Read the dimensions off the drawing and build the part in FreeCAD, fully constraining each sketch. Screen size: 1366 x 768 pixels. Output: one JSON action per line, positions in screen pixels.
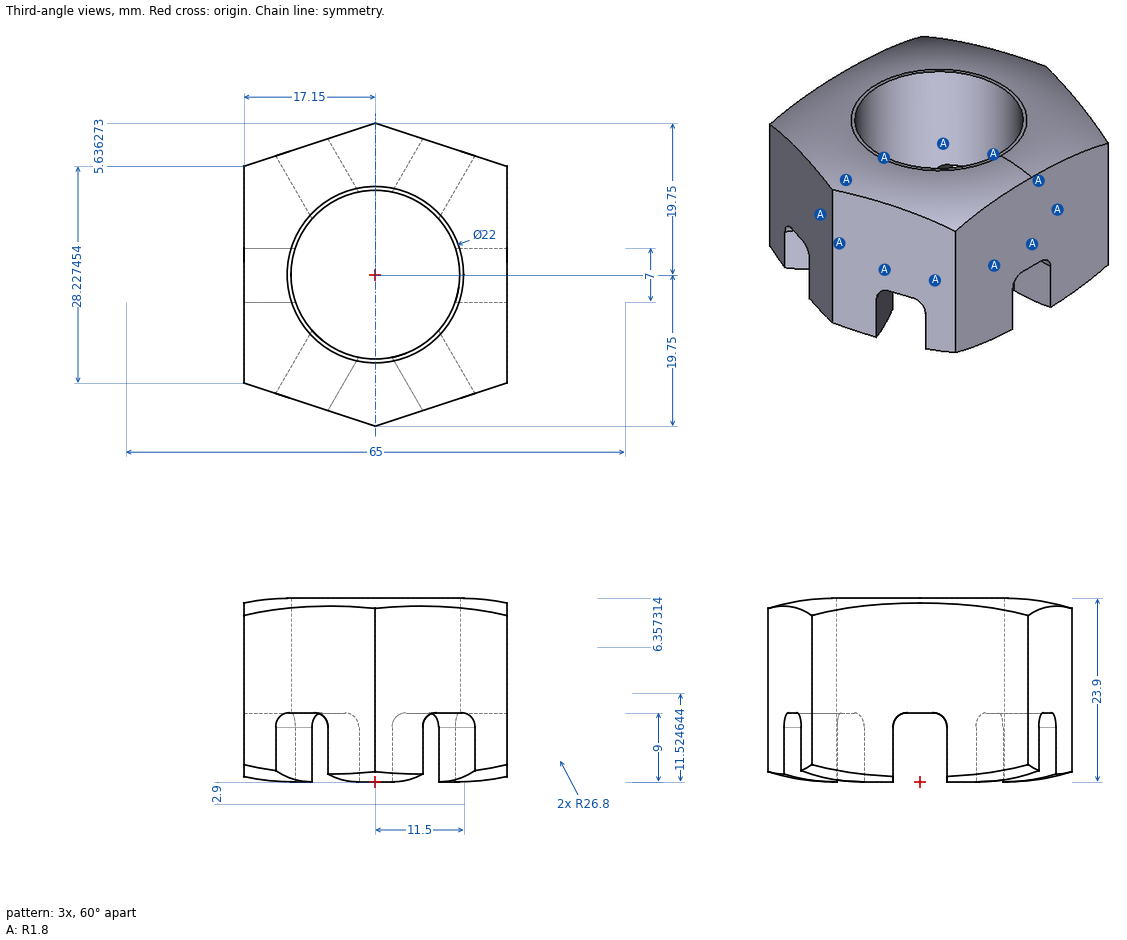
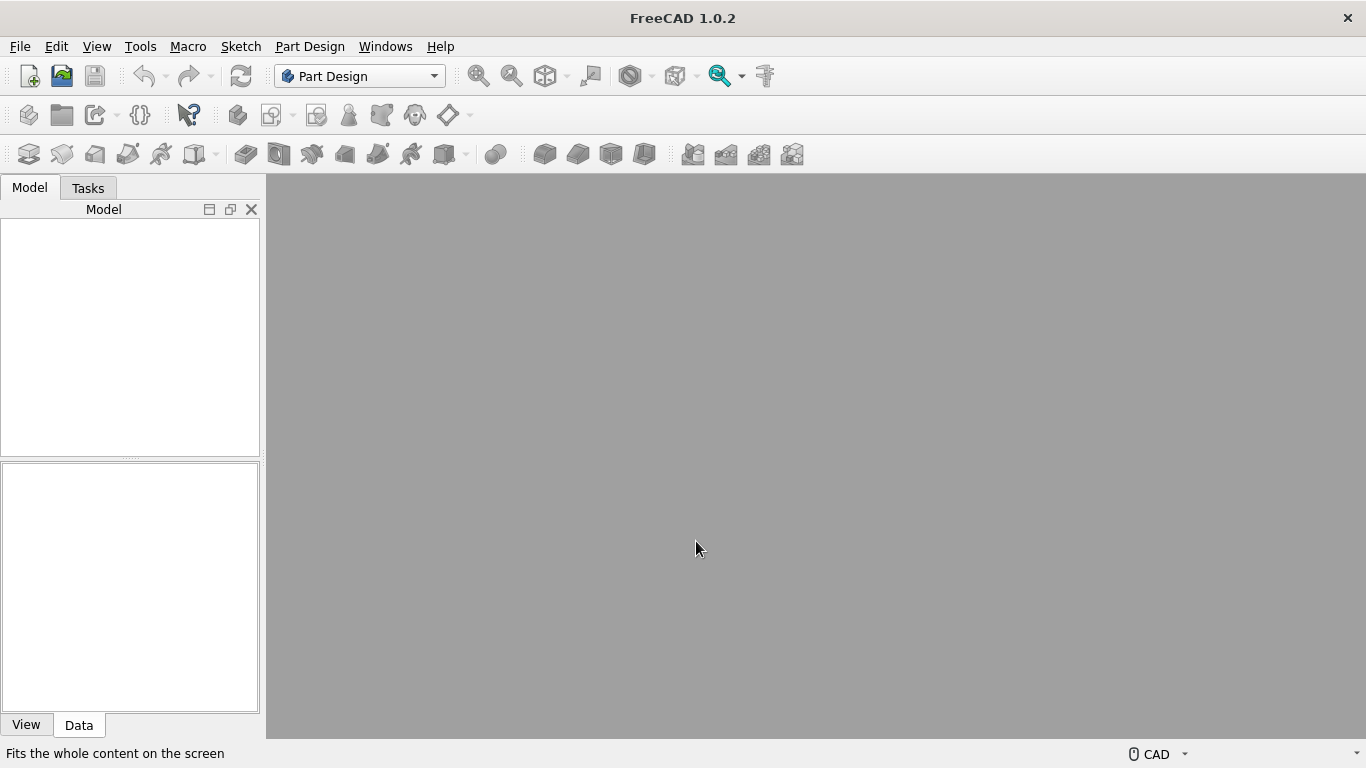
{"action": "left_click", "coordinate": [29, 76]}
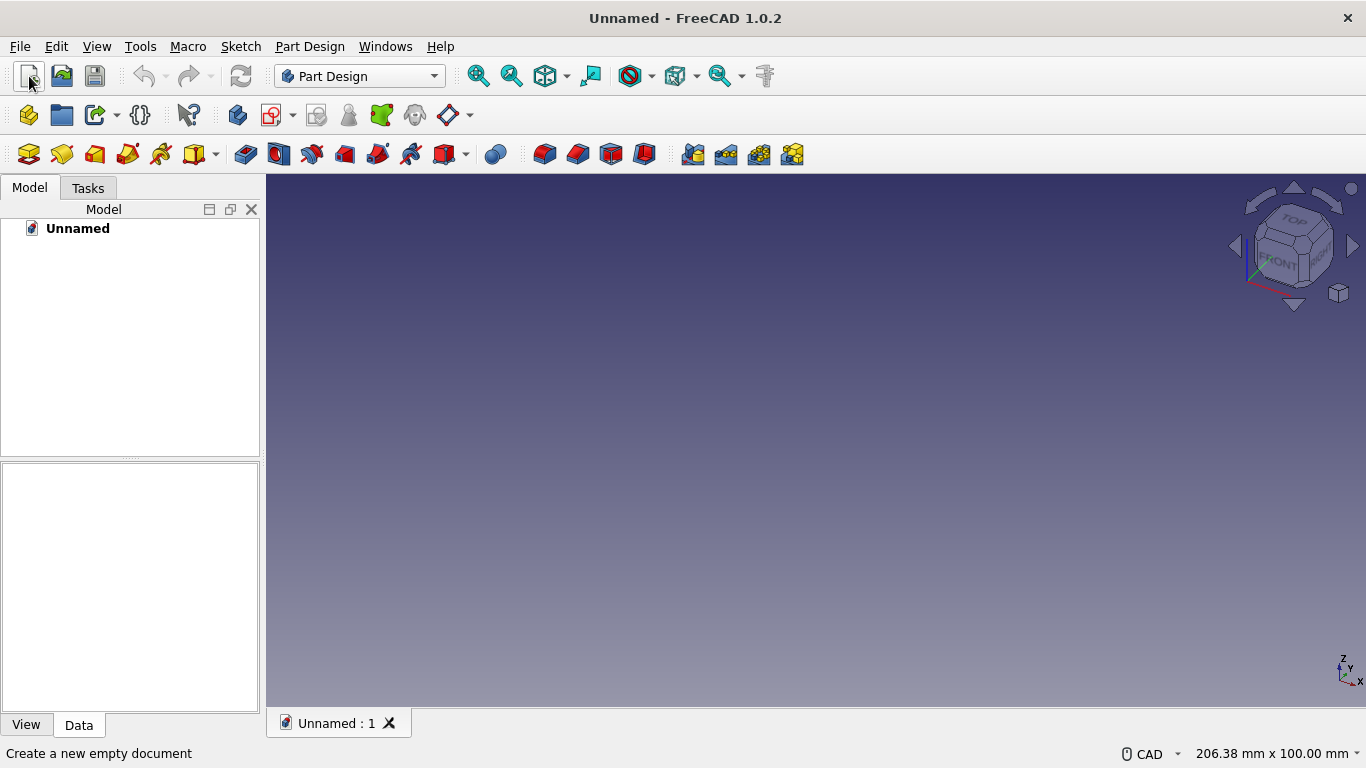
{"action": "left_click", "coordinate": [270, 116]}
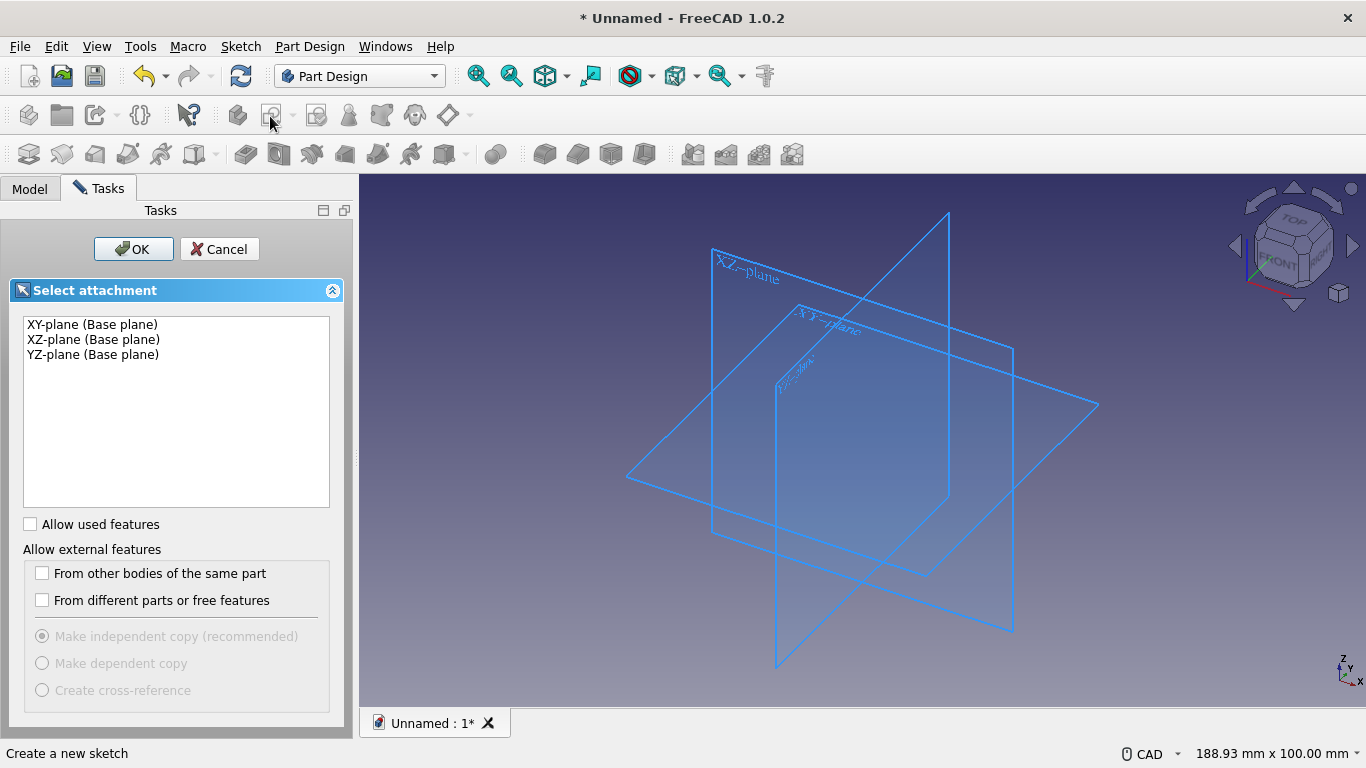
{"action": "left_click", "coordinate": [84, 324]}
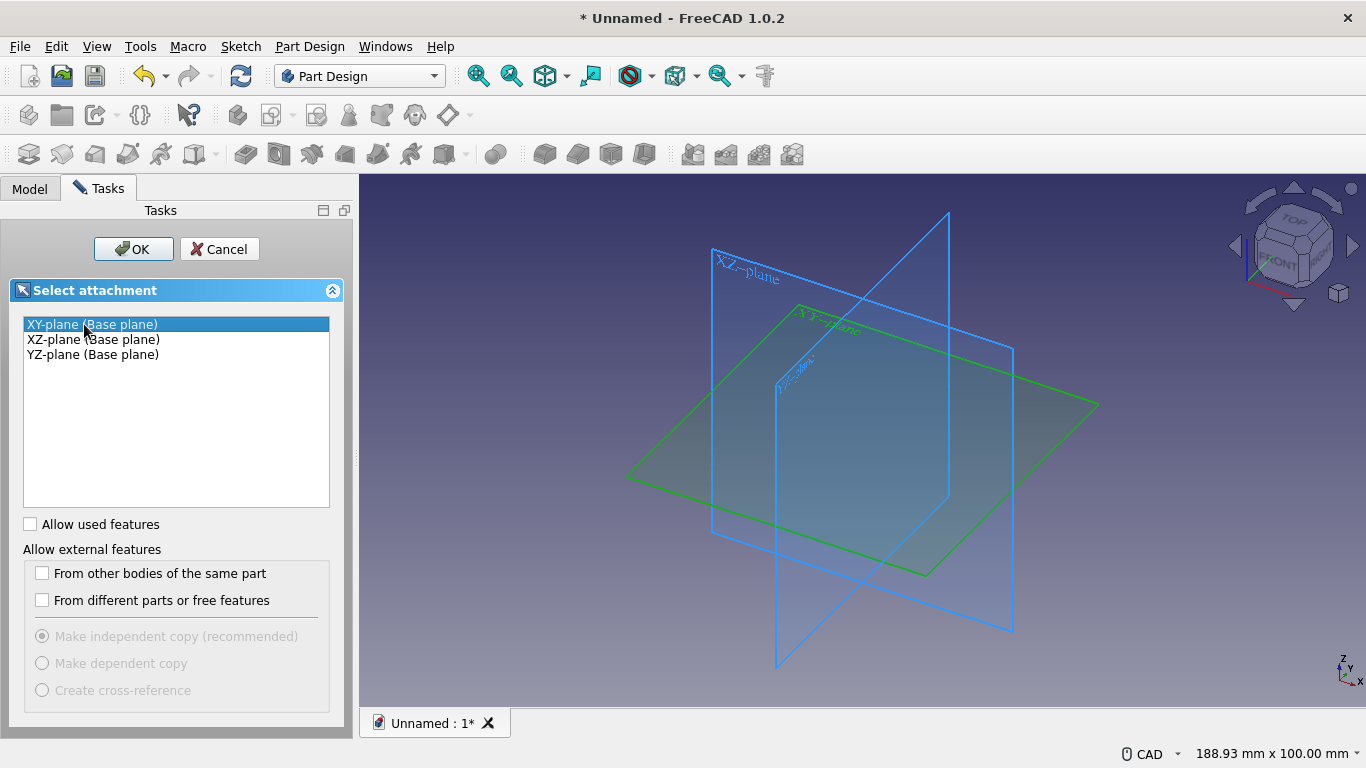
{"action": "left_click", "coordinate": [134, 249]}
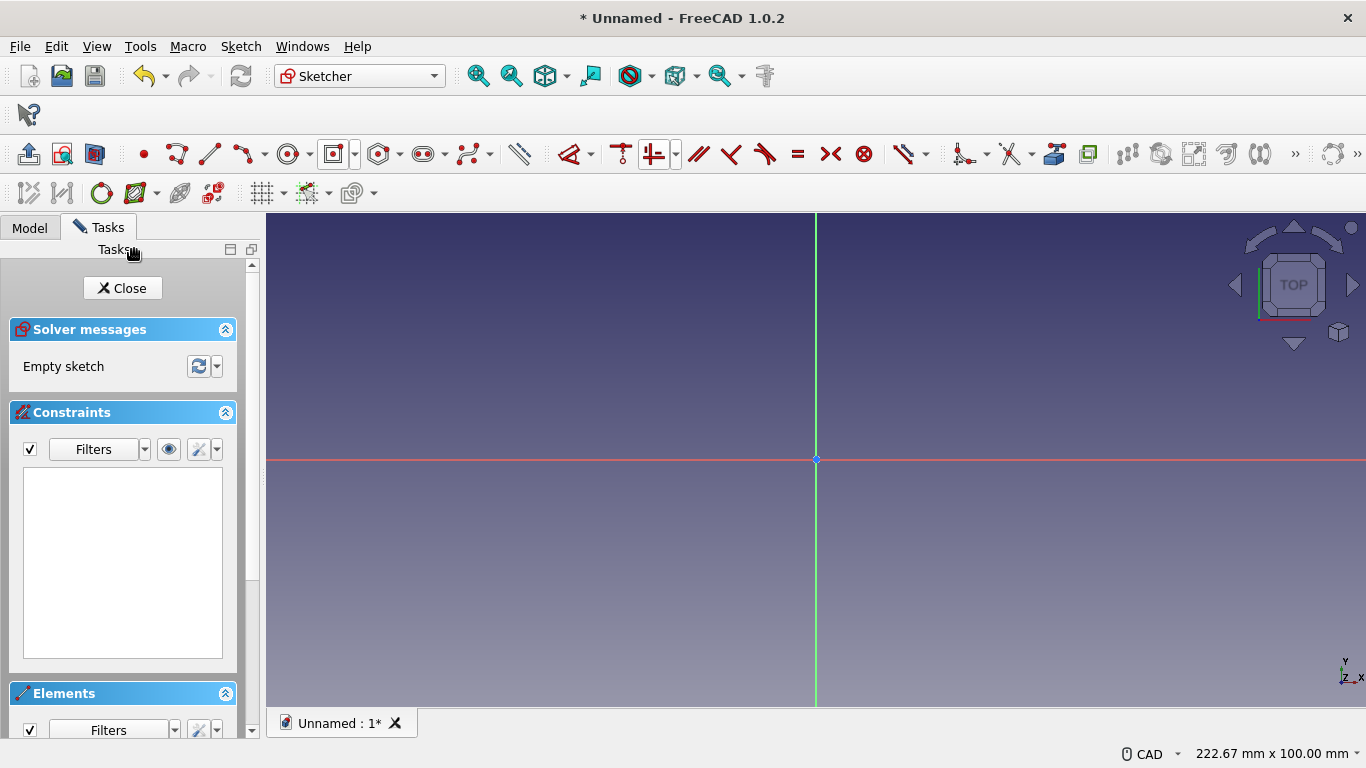
{"action": "scroll", "coordinate": [955, 460], "scroll_direction": "up", "scroll_amount": 2}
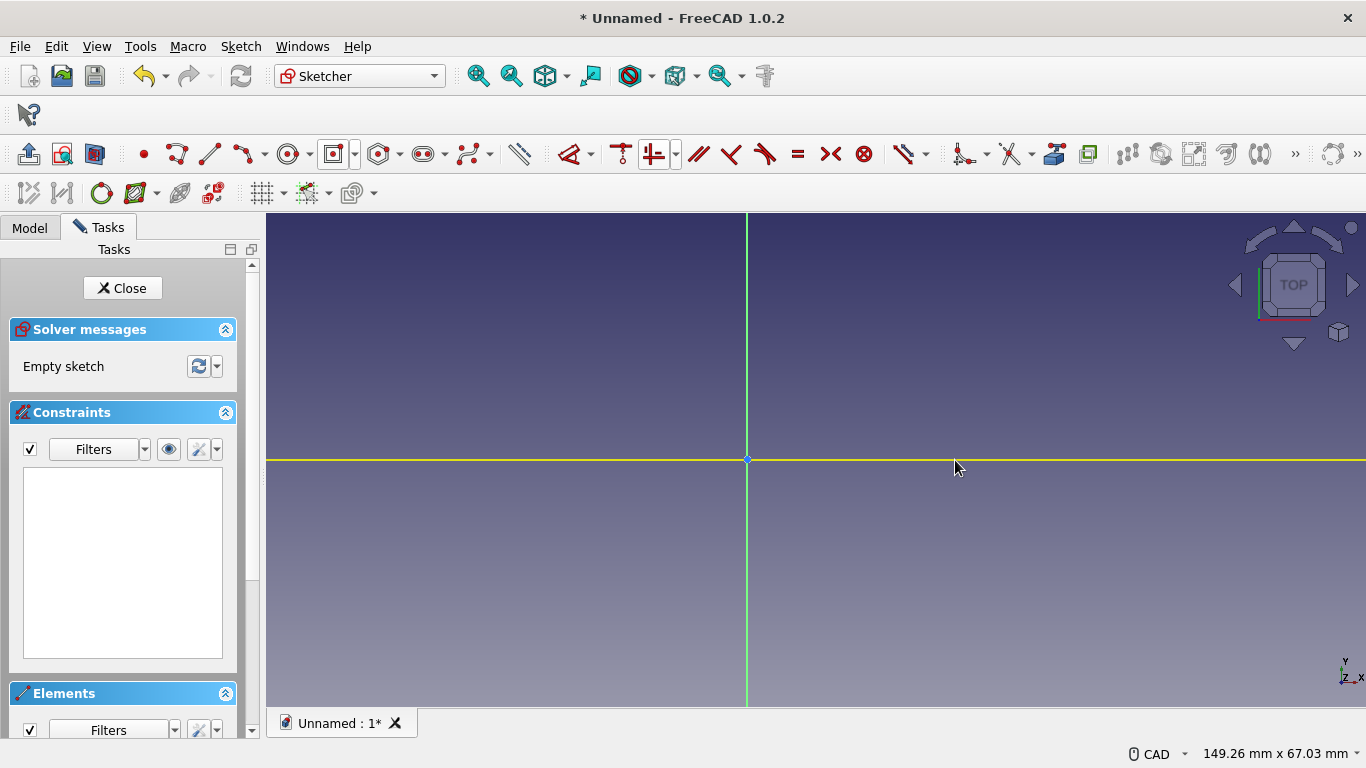
{"action": "left_click", "coordinate": [177, 154]}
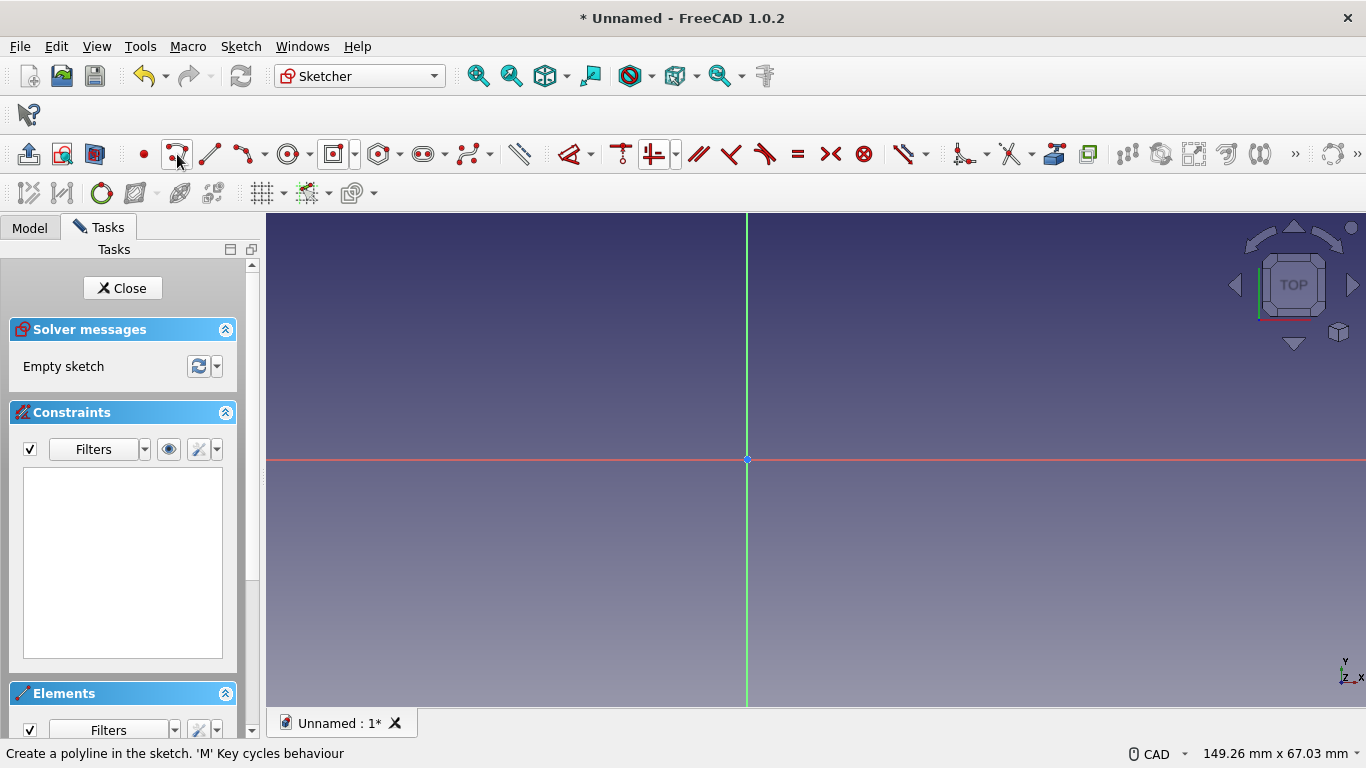
{"action": "left_click", "coordinate": [747, 314]}
{"action": "left_click", "coordinate": [621, 356]}
{"action": "left_click", "coordinate": [621, 564]}
{"action": "left_click", "coordinate": [747, 605]}
{"action": "left_click", "coordinate": [874, 564]}
{"action": "left_click", "coordinate": [874, 356]}
{"action": "left_click", "coordinate": [747, 315]}
{"action": "key", "text": "Escape"}
{"action": "key", "text": "Escape"}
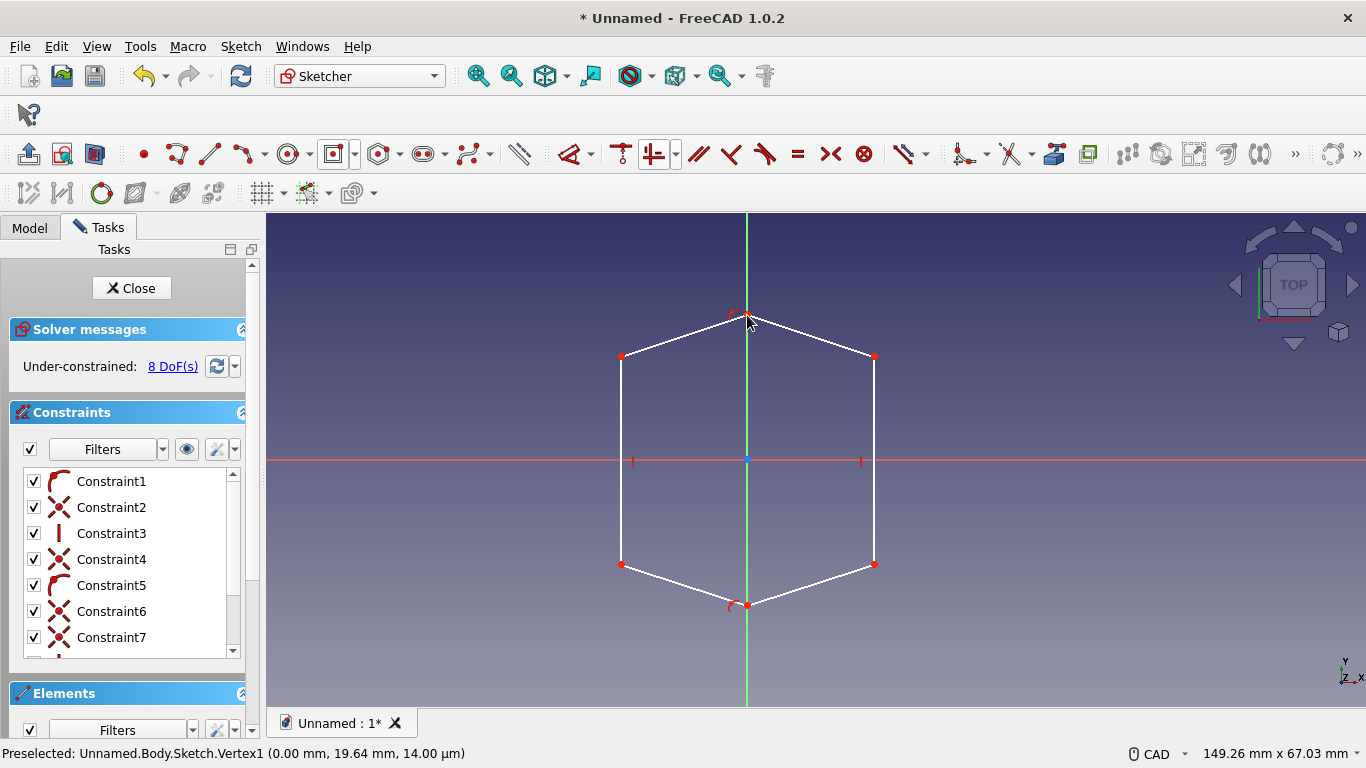
{"action": "left_click", "coordinate": [621, 565]}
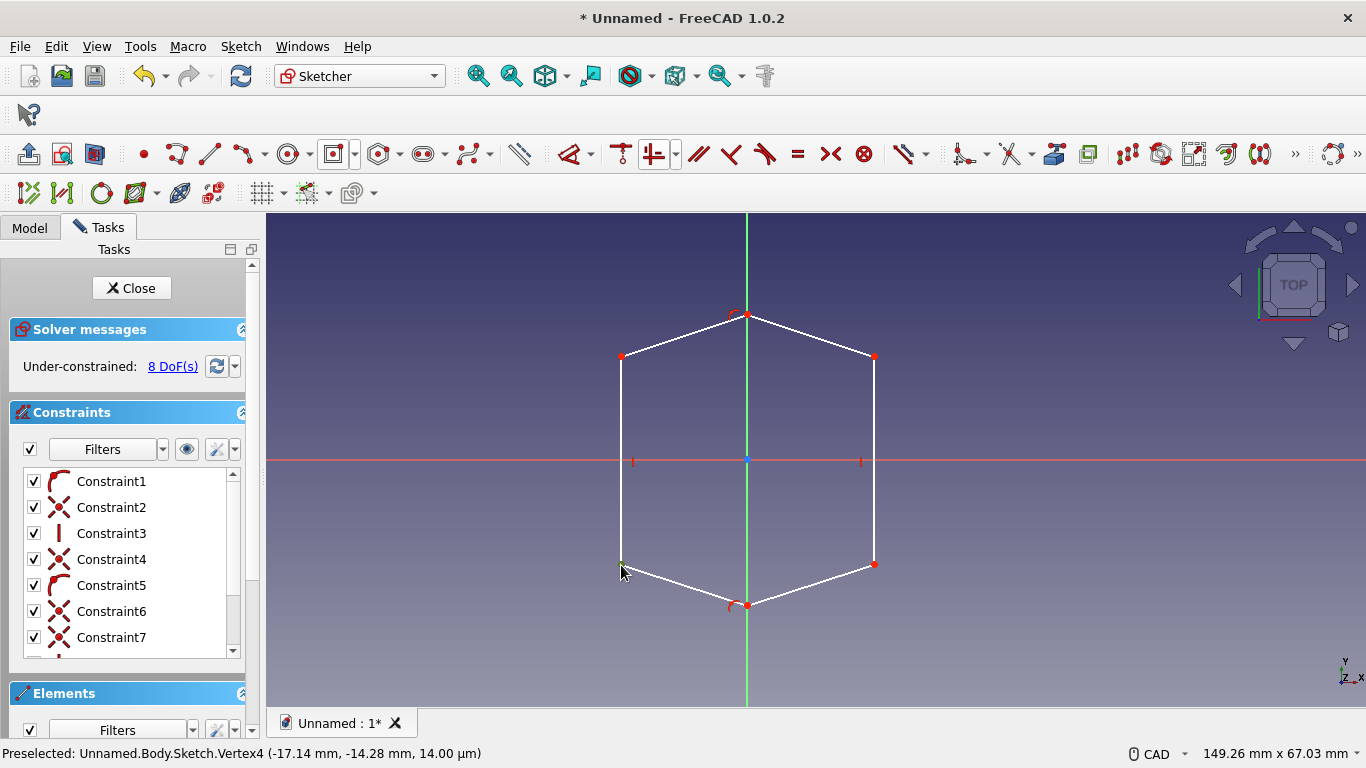
{"action": "left_click", "coordinate": [874, 565]}